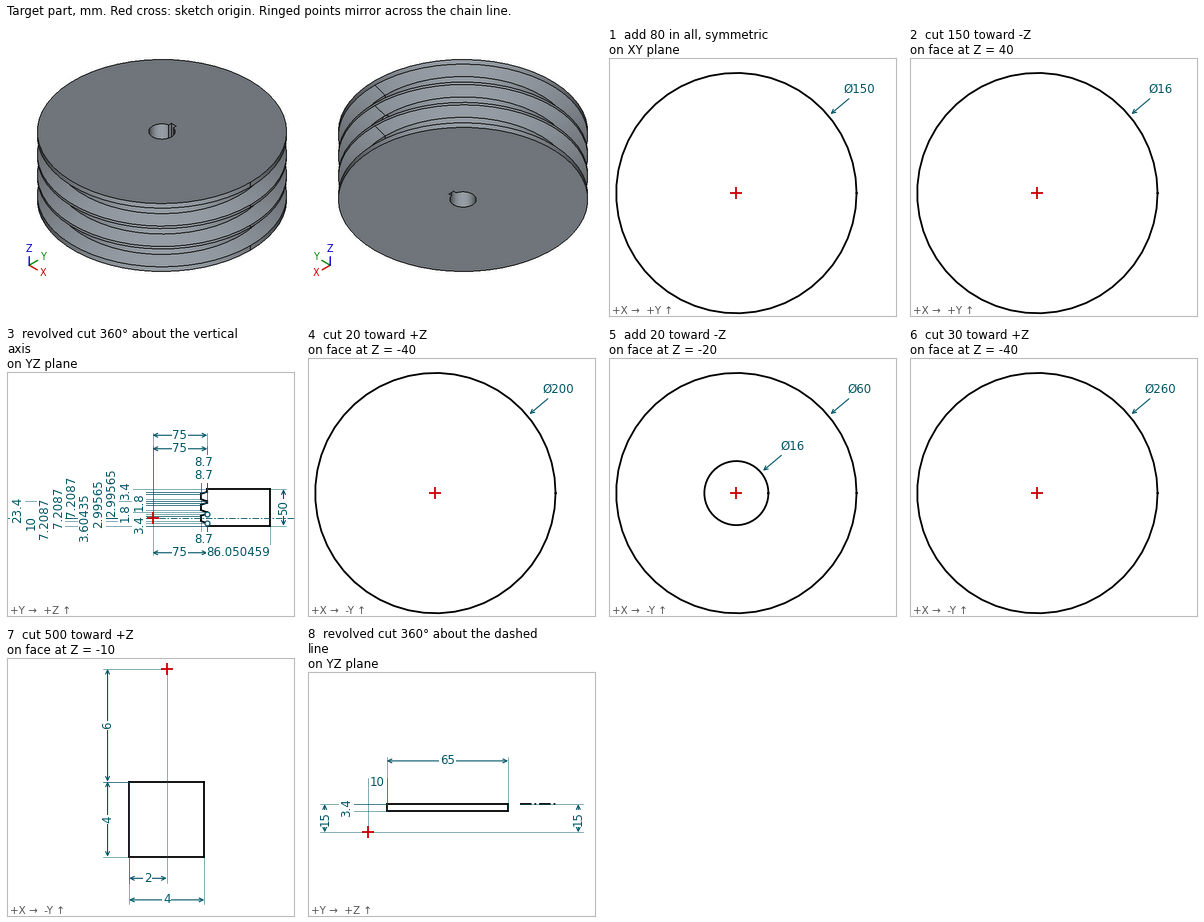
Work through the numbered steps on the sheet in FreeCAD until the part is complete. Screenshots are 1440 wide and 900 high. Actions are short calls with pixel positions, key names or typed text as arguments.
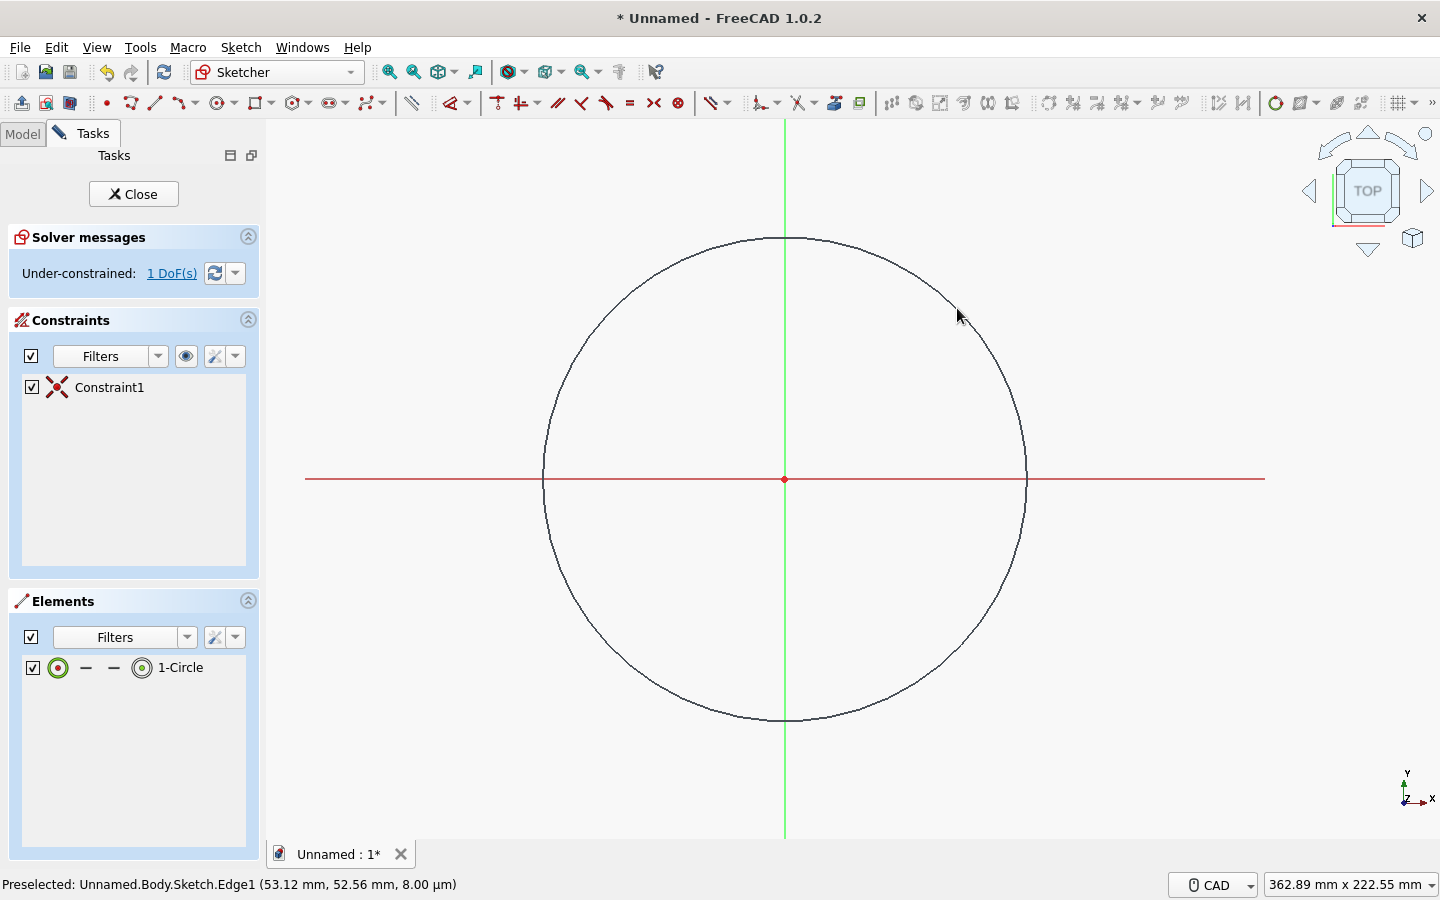
click(450, 104)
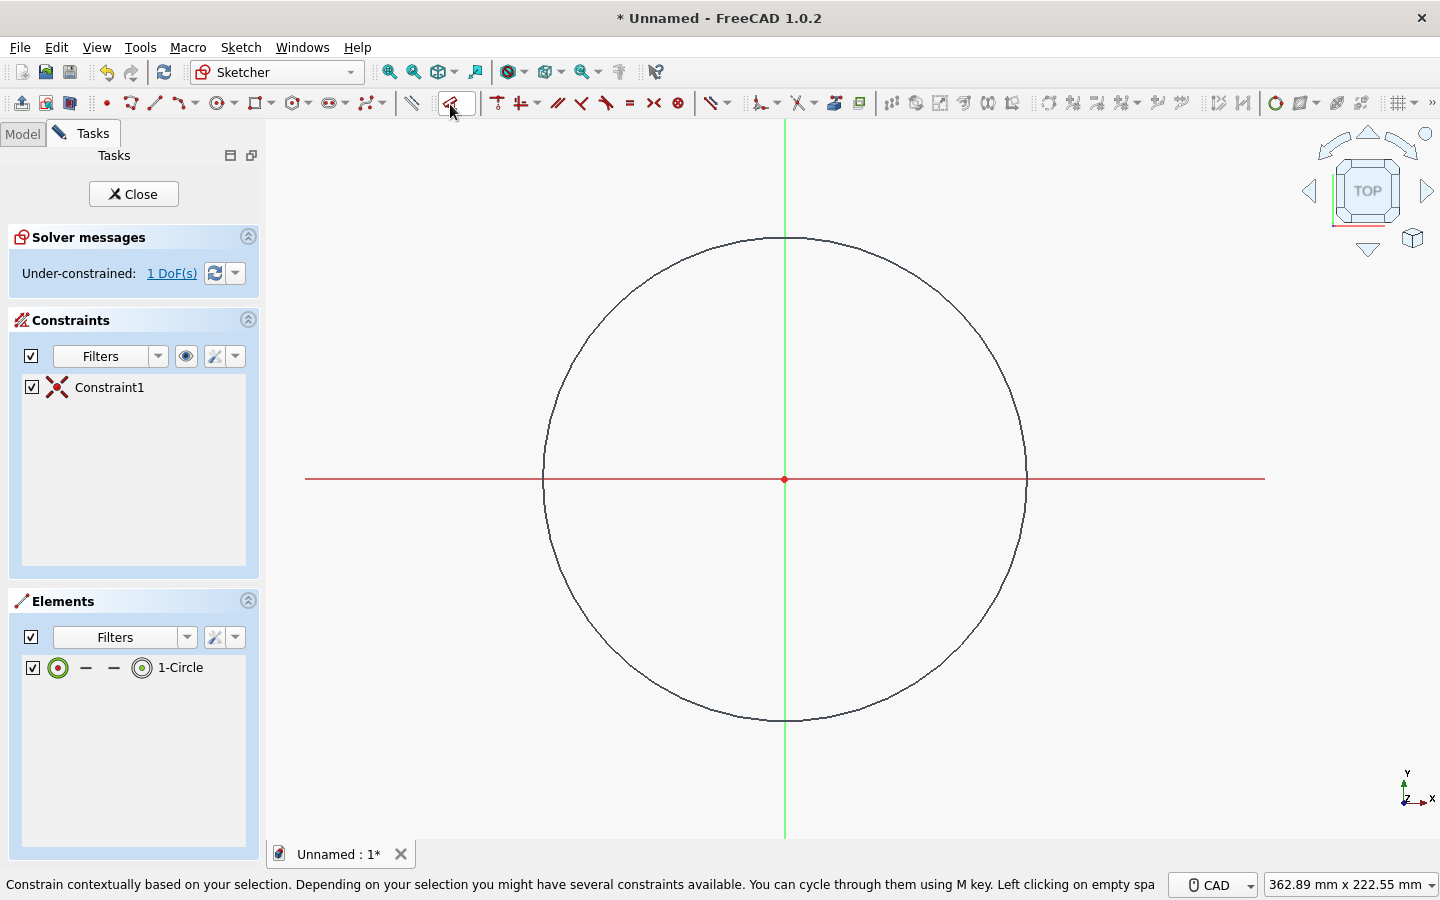
click(956, 308)
click(979, 285)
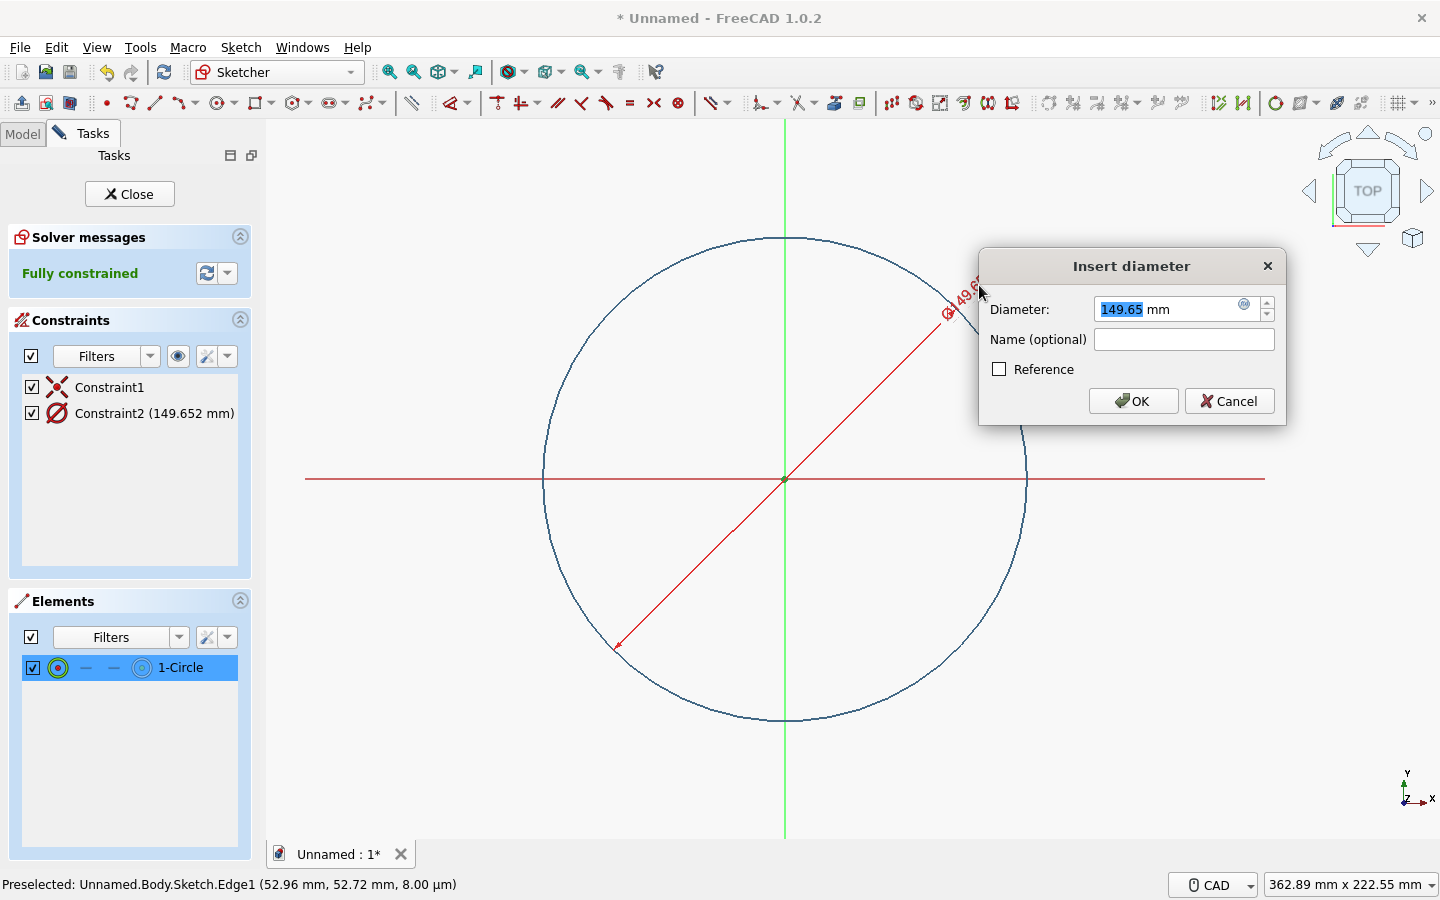
text(150)
key(Return)
key(Escape)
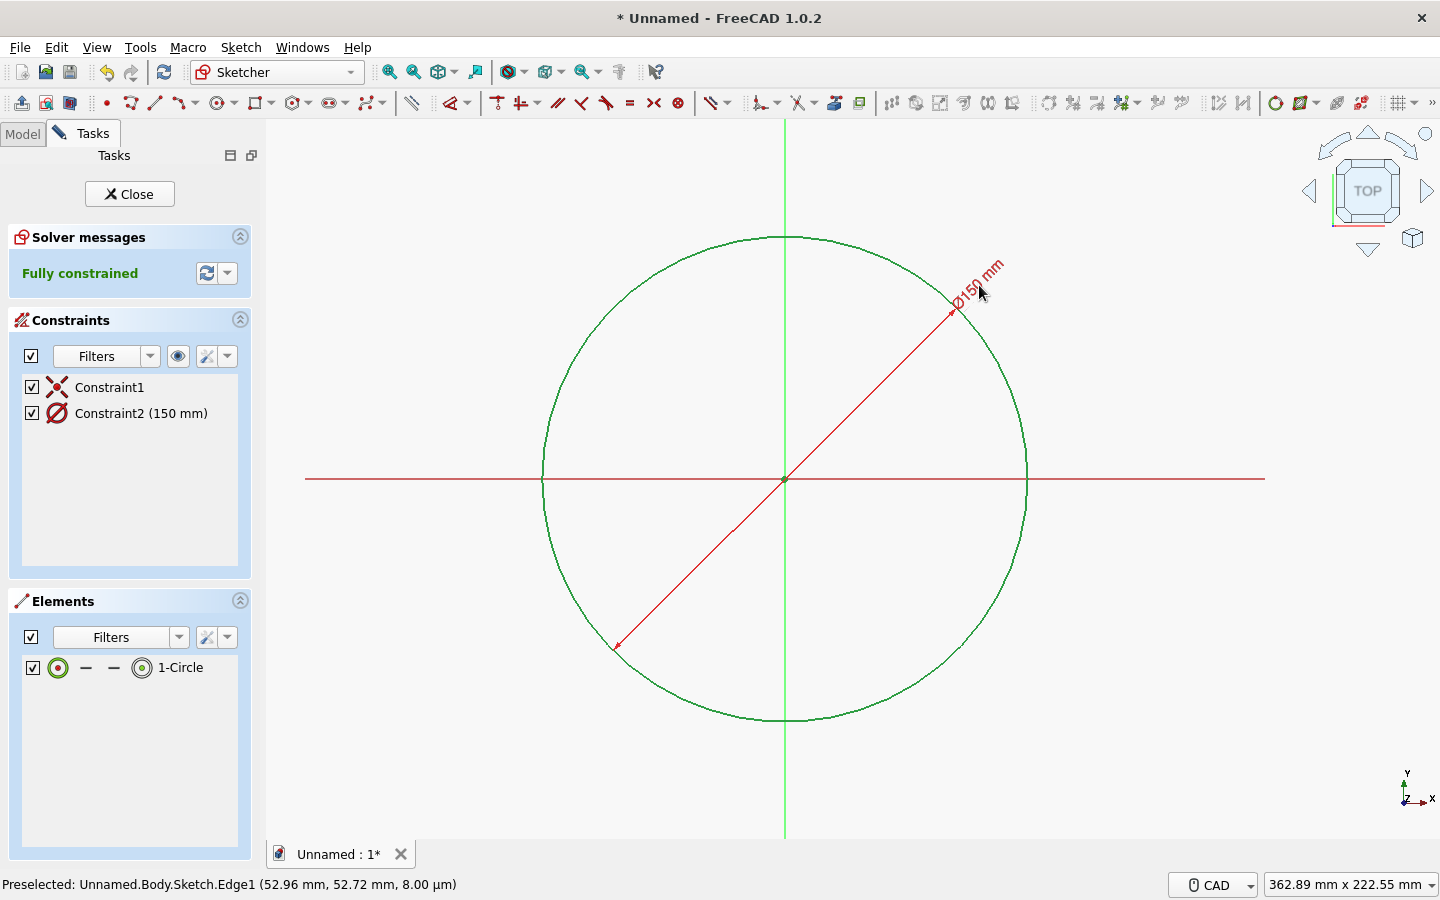
click(130, 194)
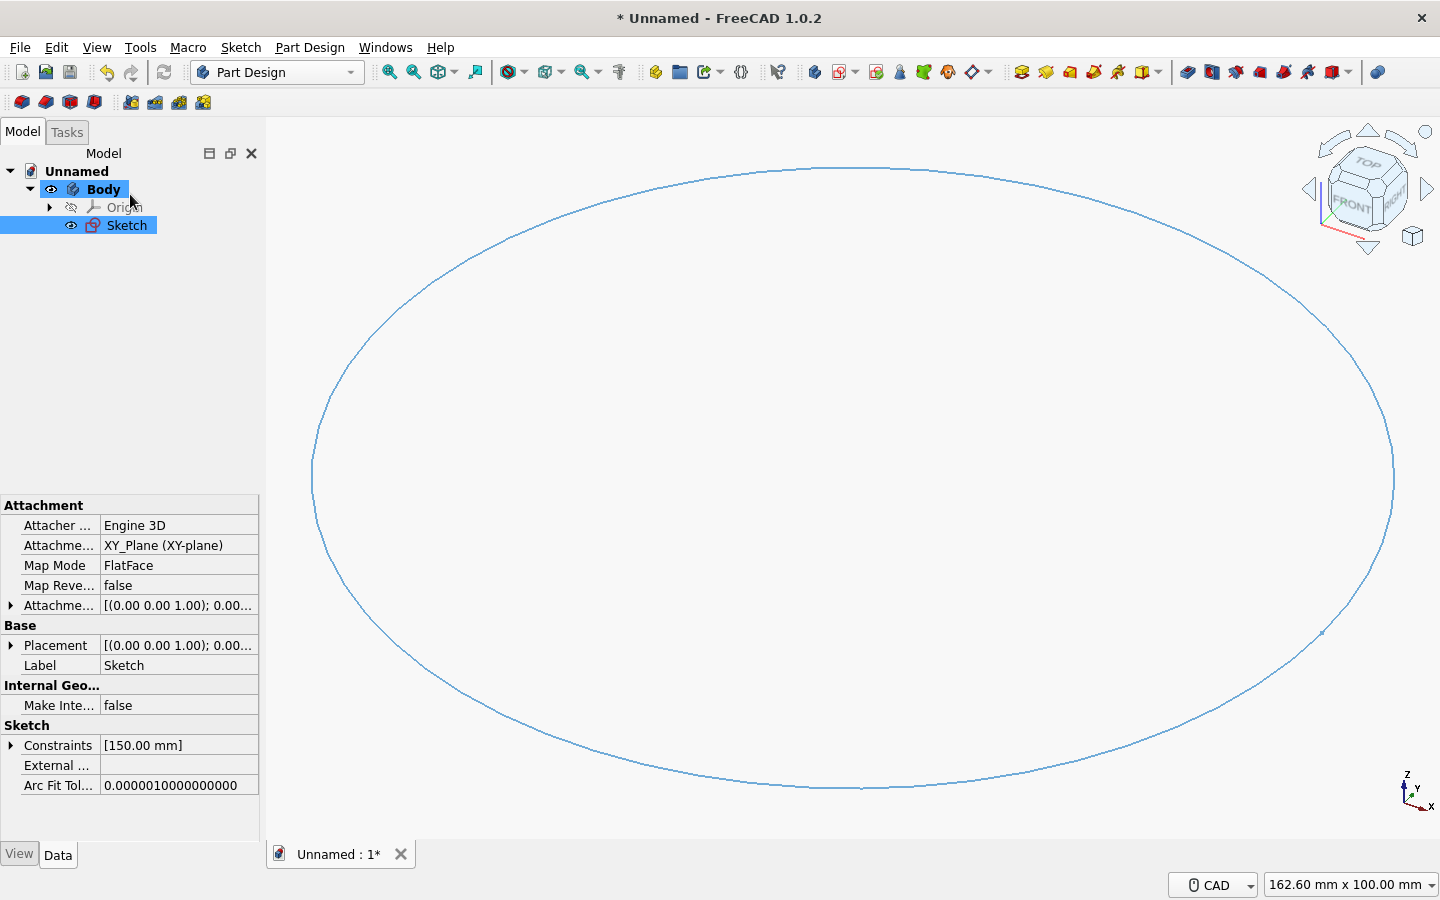
click(1022, 72)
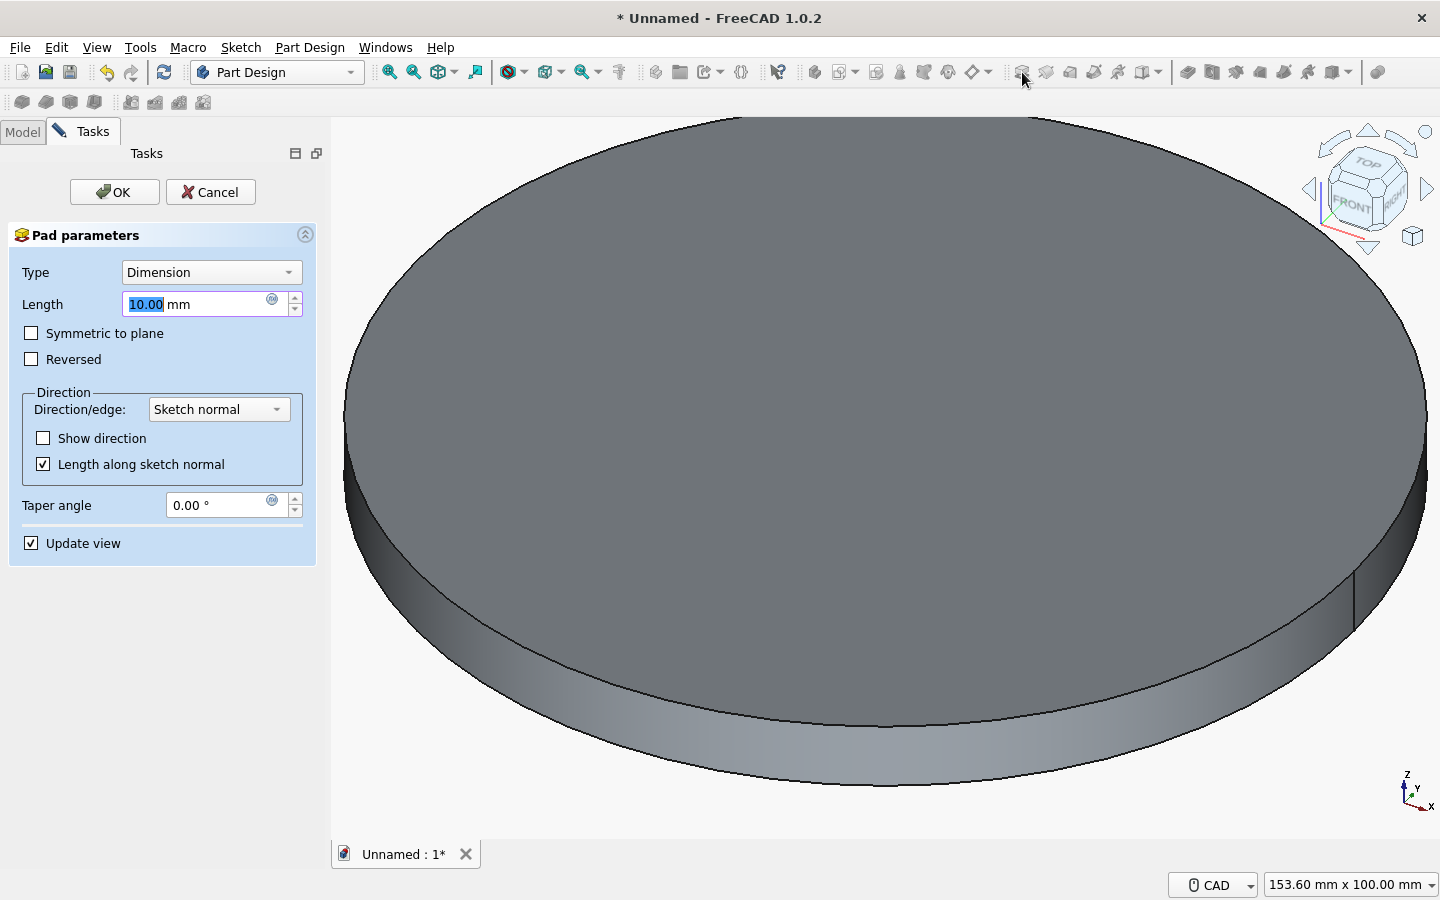
text(80)
key(Tab)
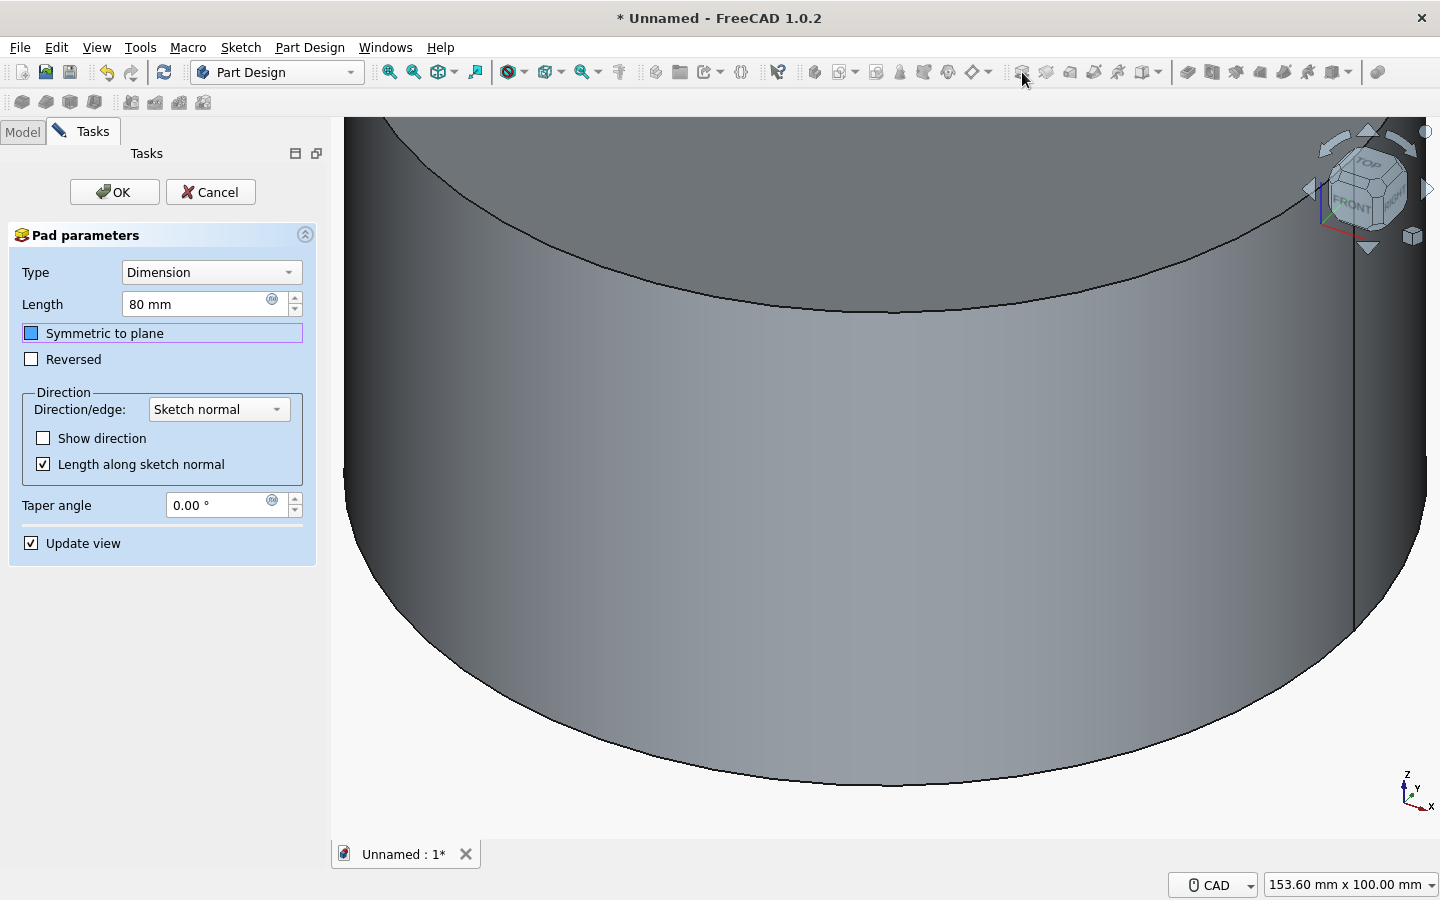
click(30, 333)